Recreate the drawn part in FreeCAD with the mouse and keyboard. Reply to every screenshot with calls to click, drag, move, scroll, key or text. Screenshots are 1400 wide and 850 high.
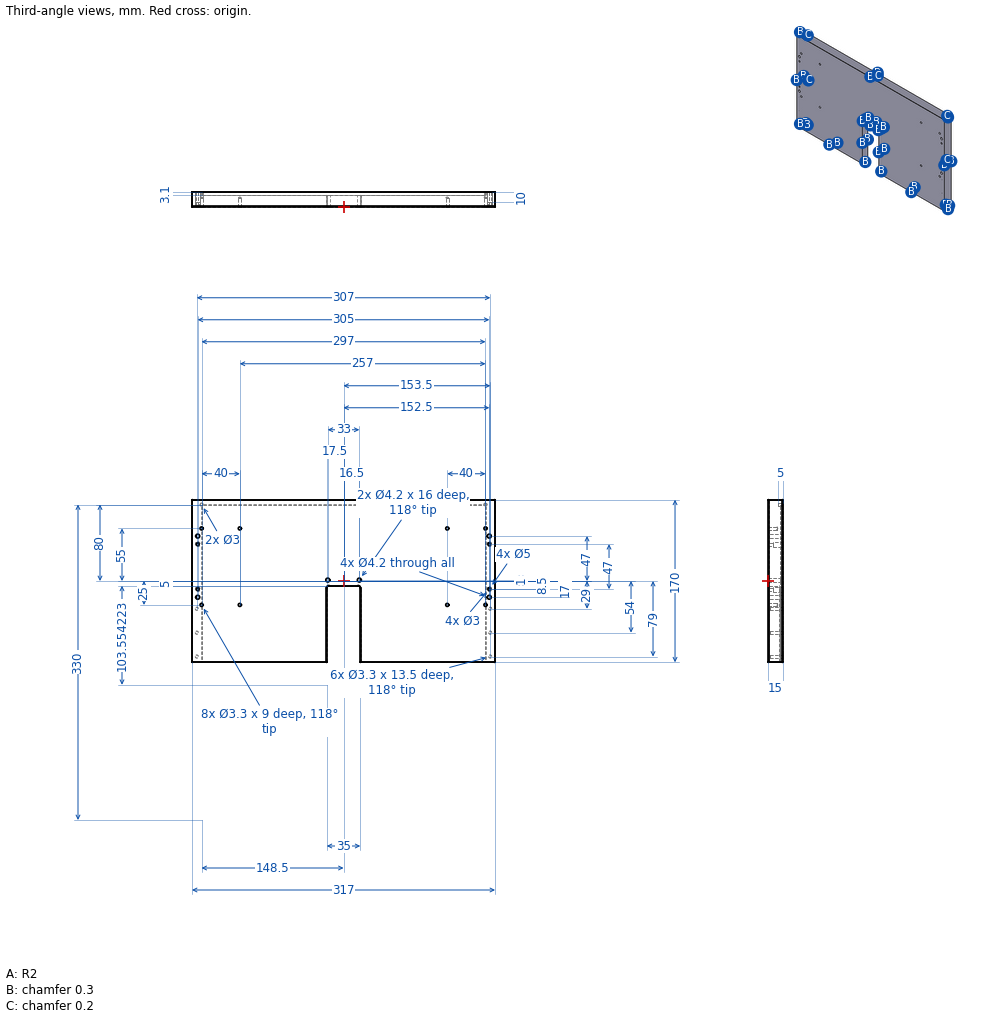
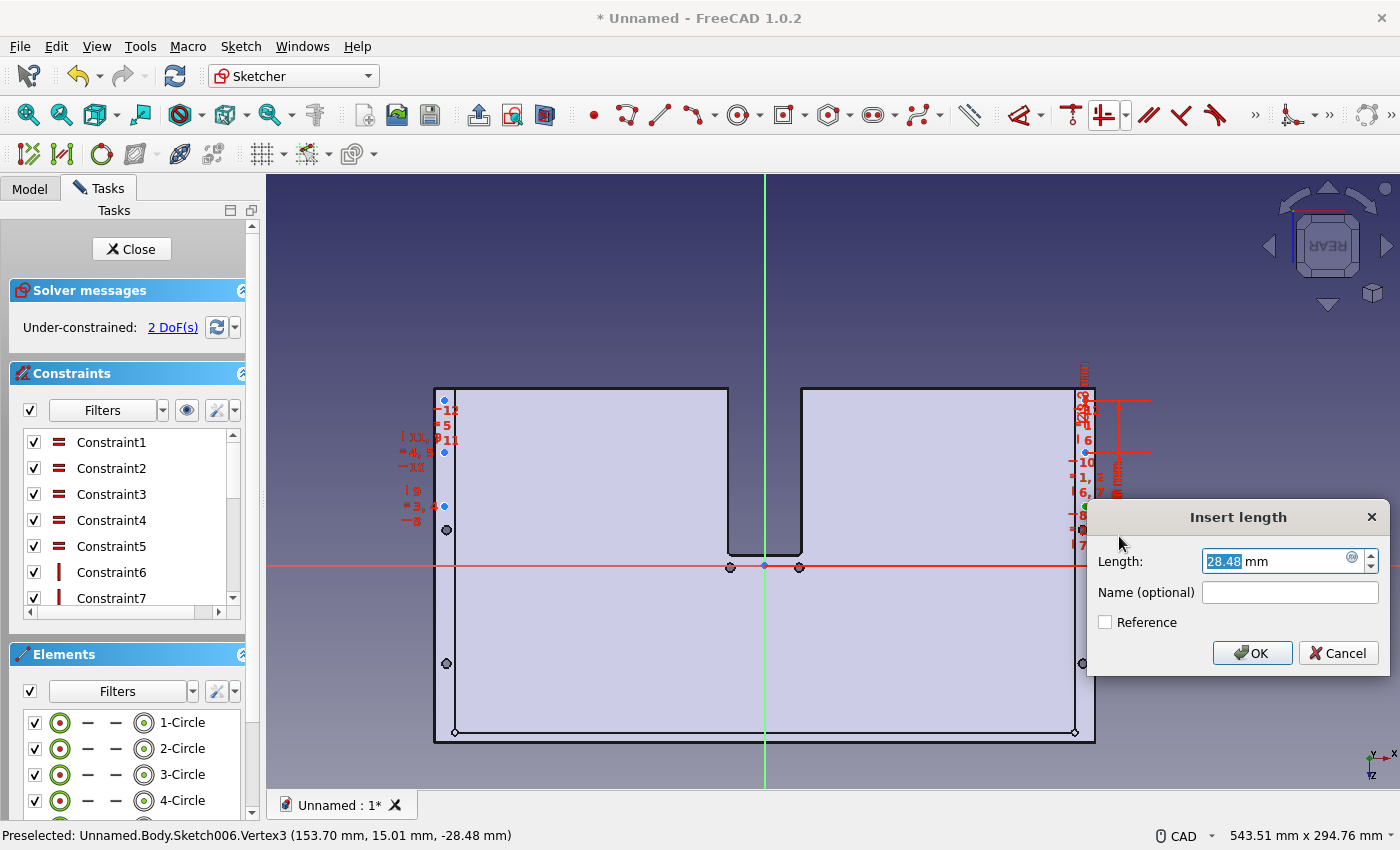
text(29)
key(Return)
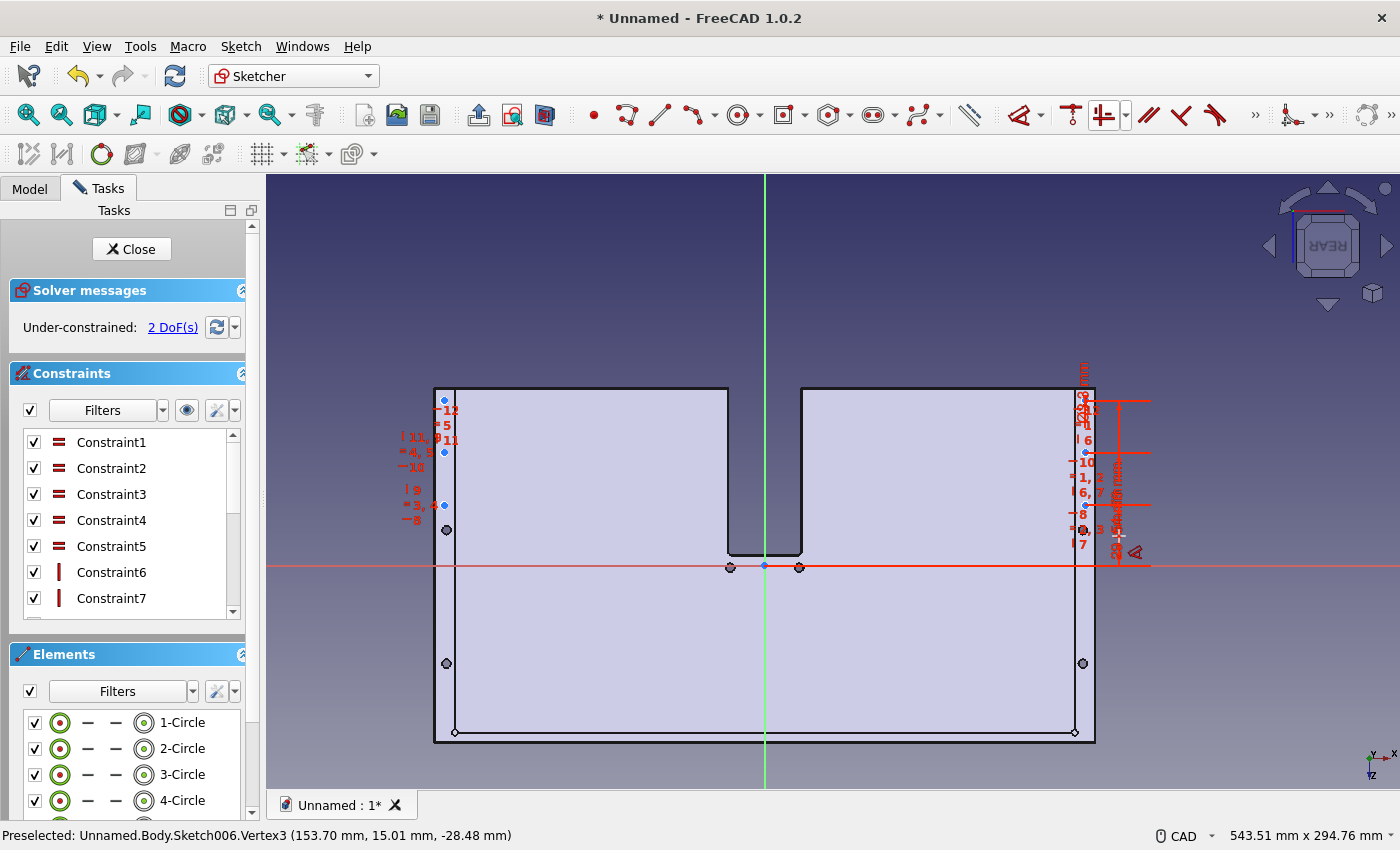
click(1085, 505)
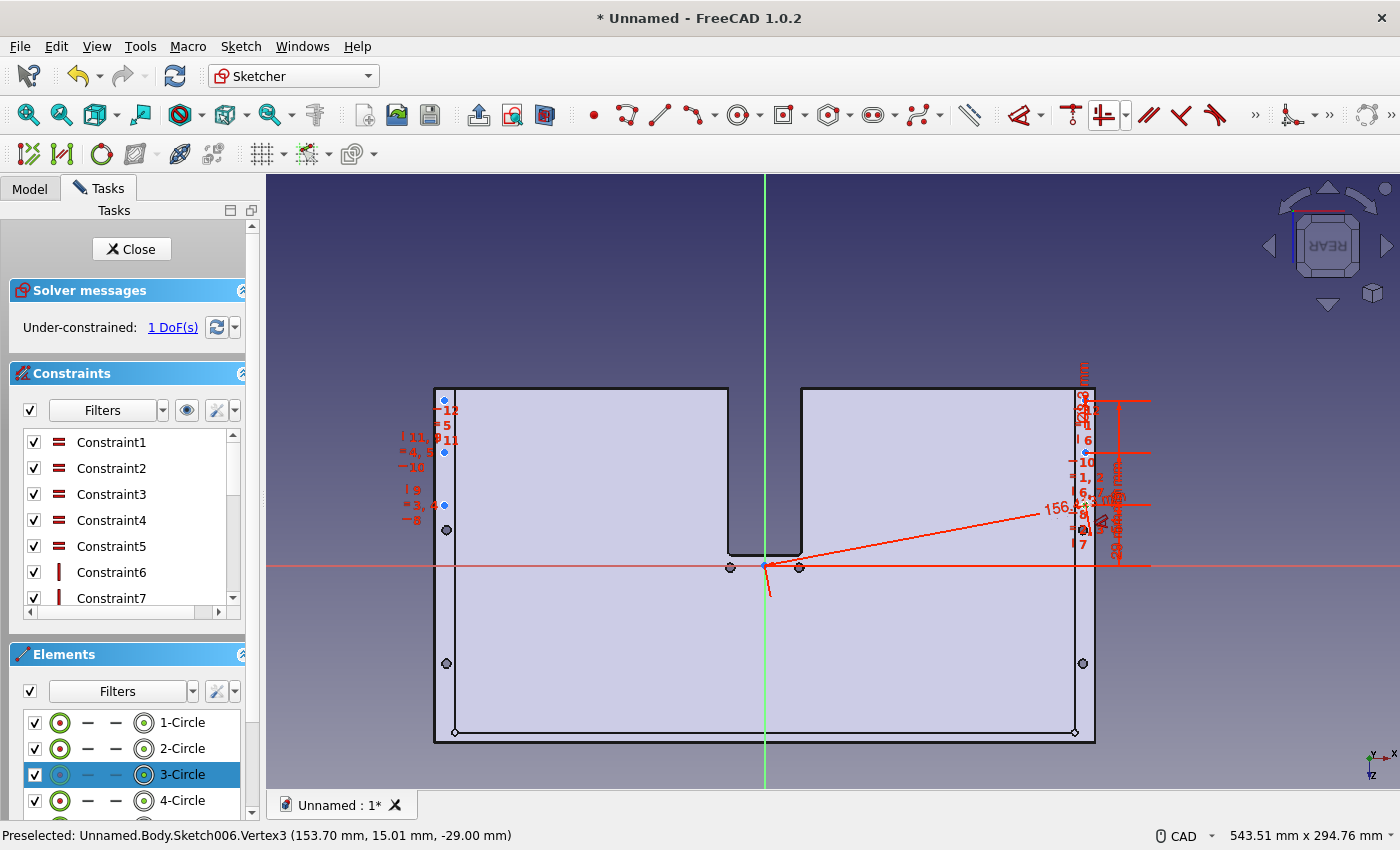
click(444, 505)
click(617, 539)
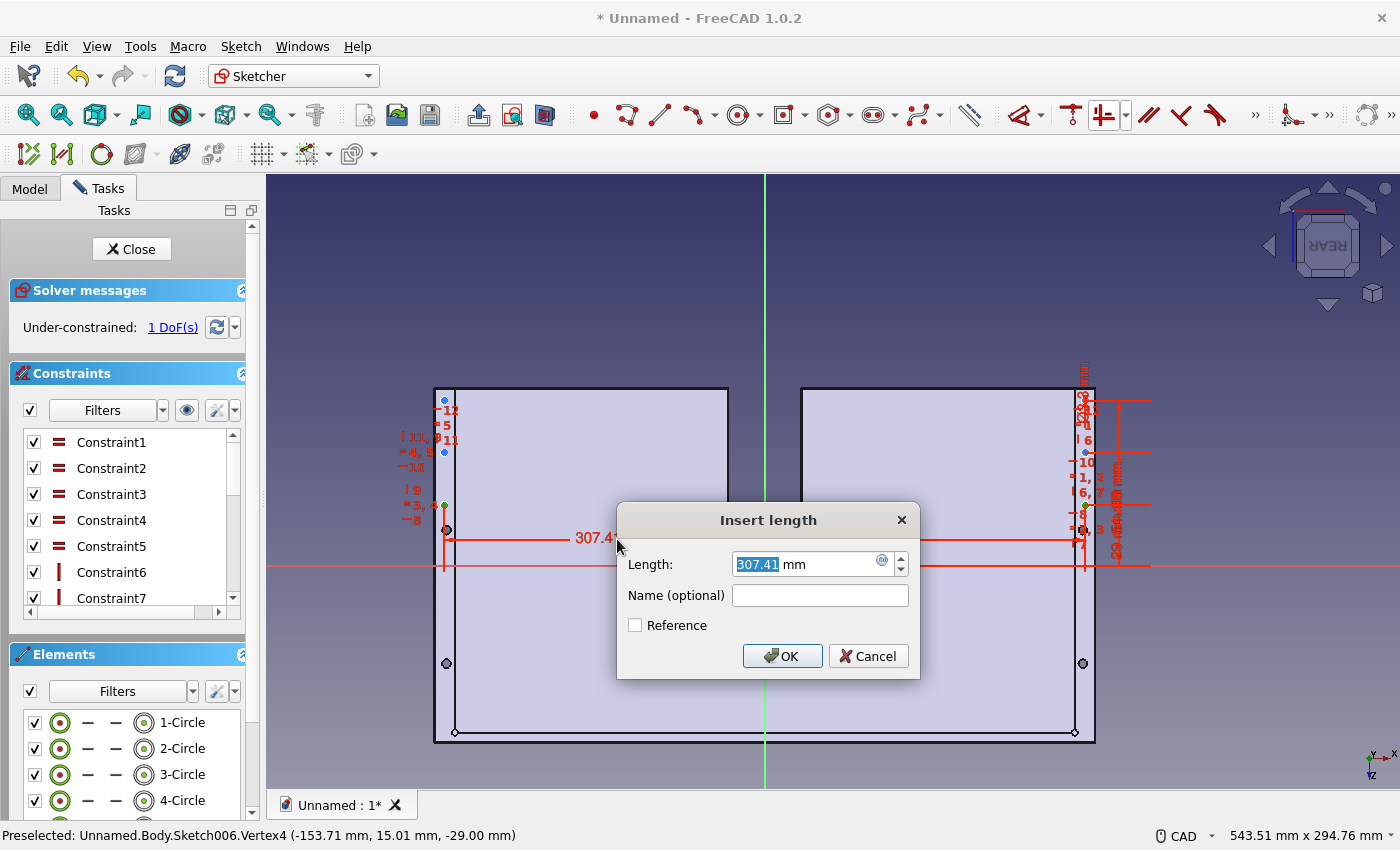
text(307)
key(Return)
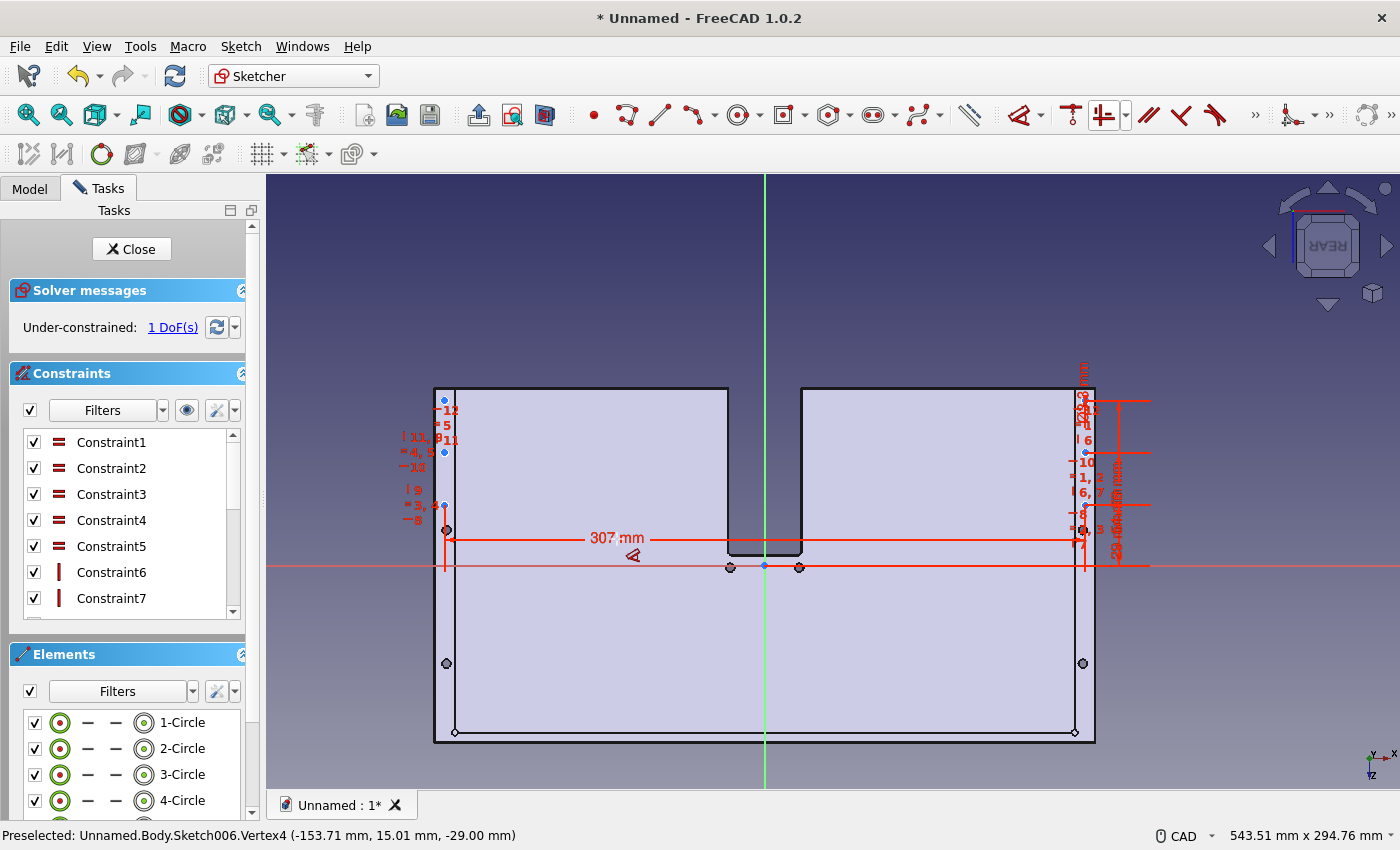
click(1085, 401)
click(925, 600)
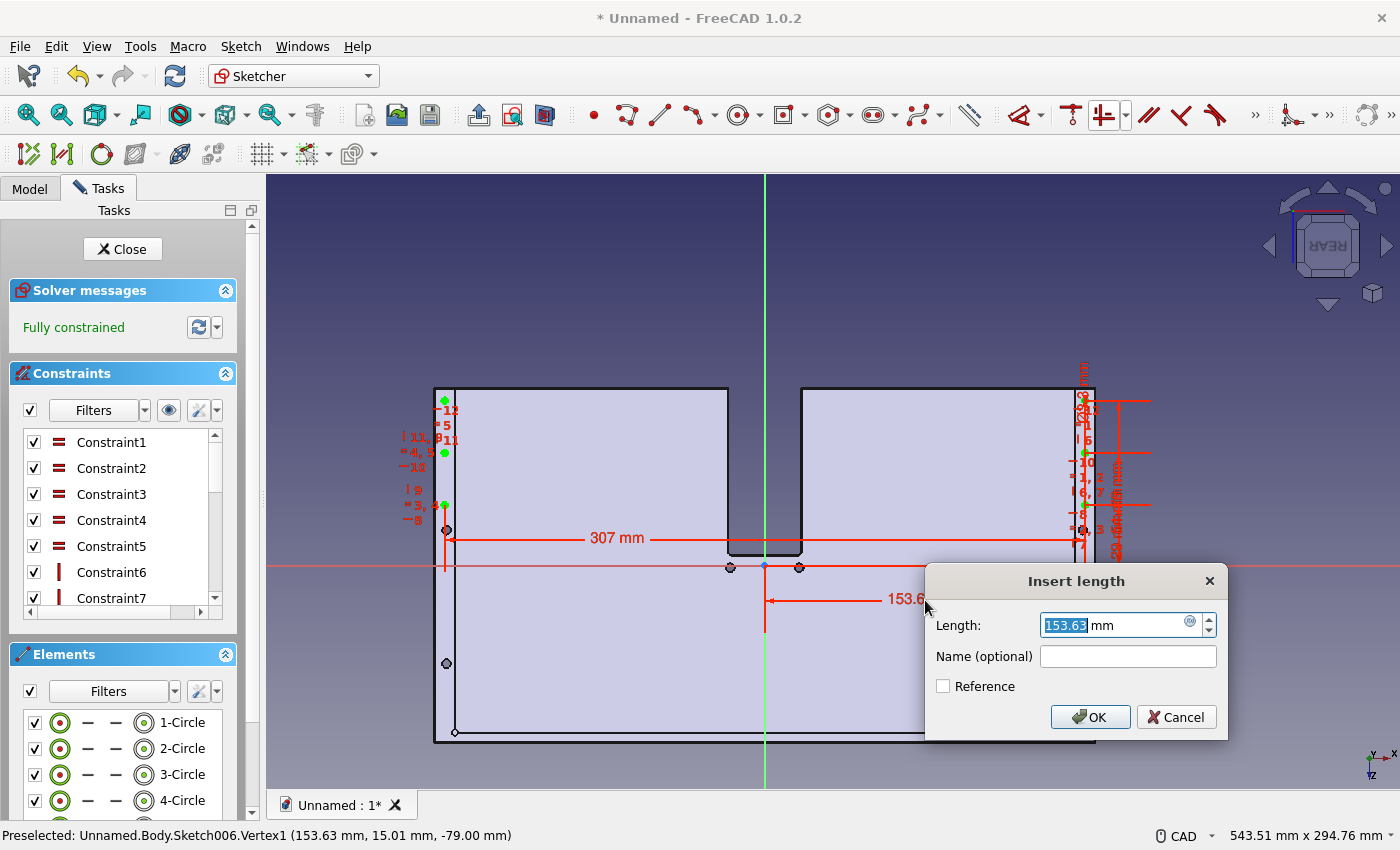
text(153.5)
key(Return)
key(Escape)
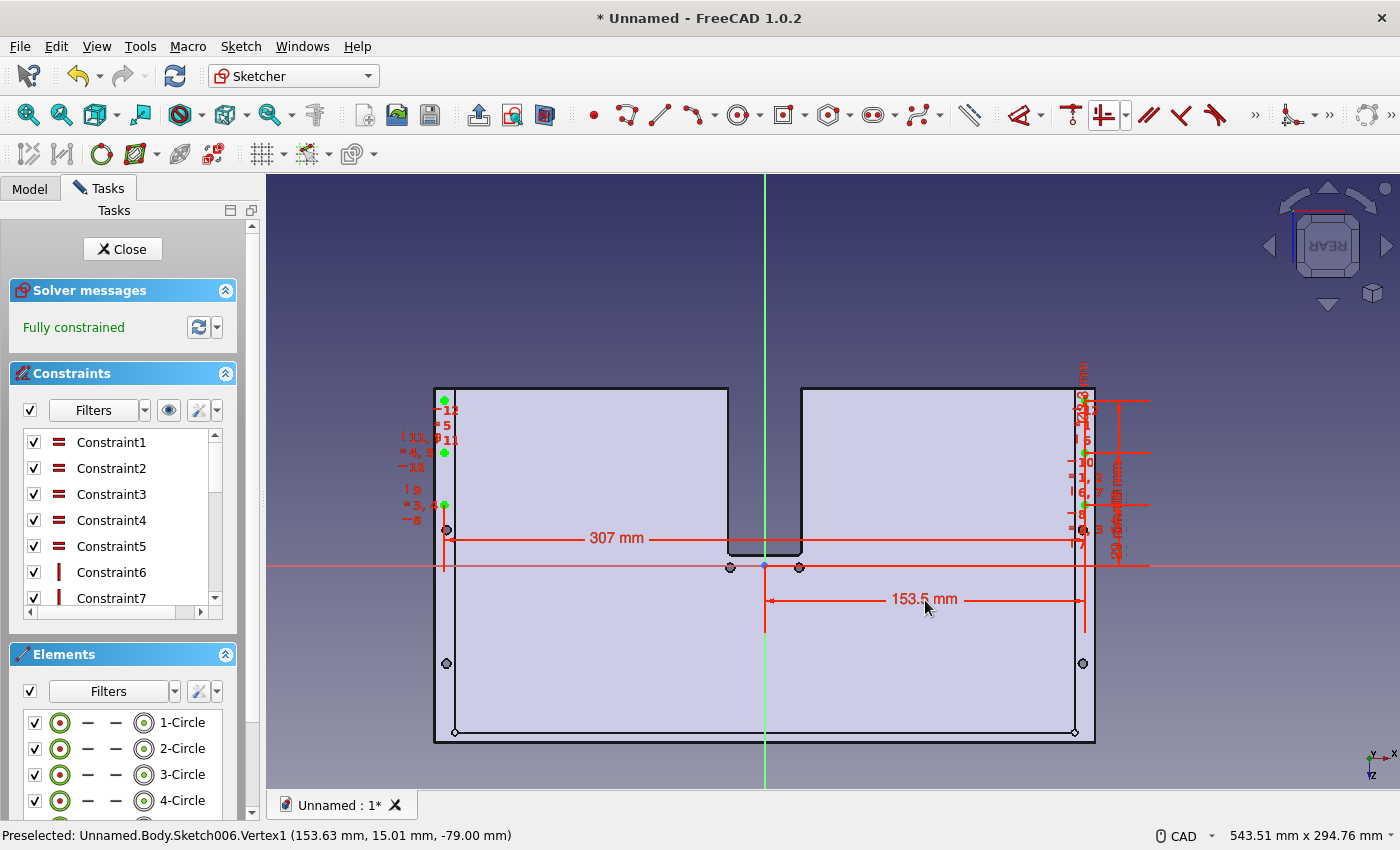
click(123, 249)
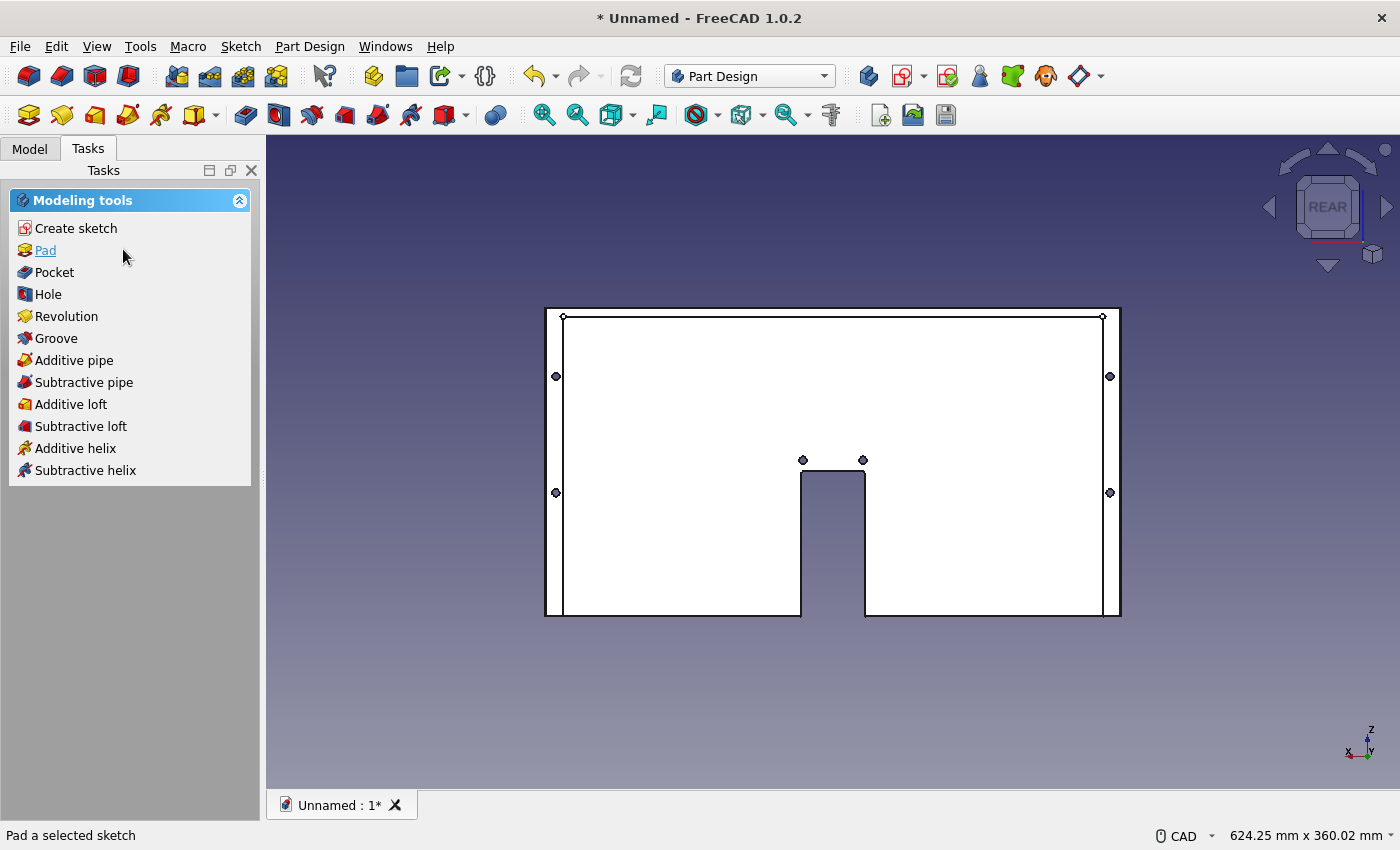
click(279, 116)